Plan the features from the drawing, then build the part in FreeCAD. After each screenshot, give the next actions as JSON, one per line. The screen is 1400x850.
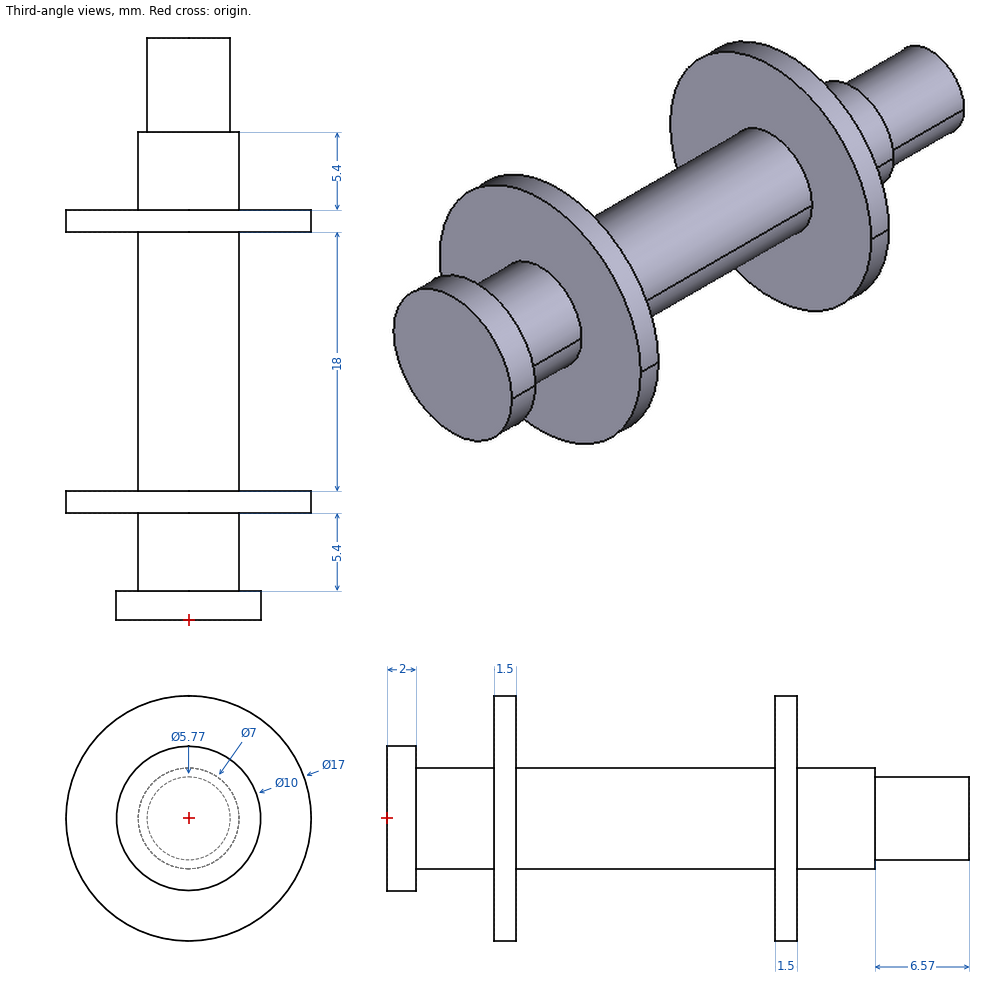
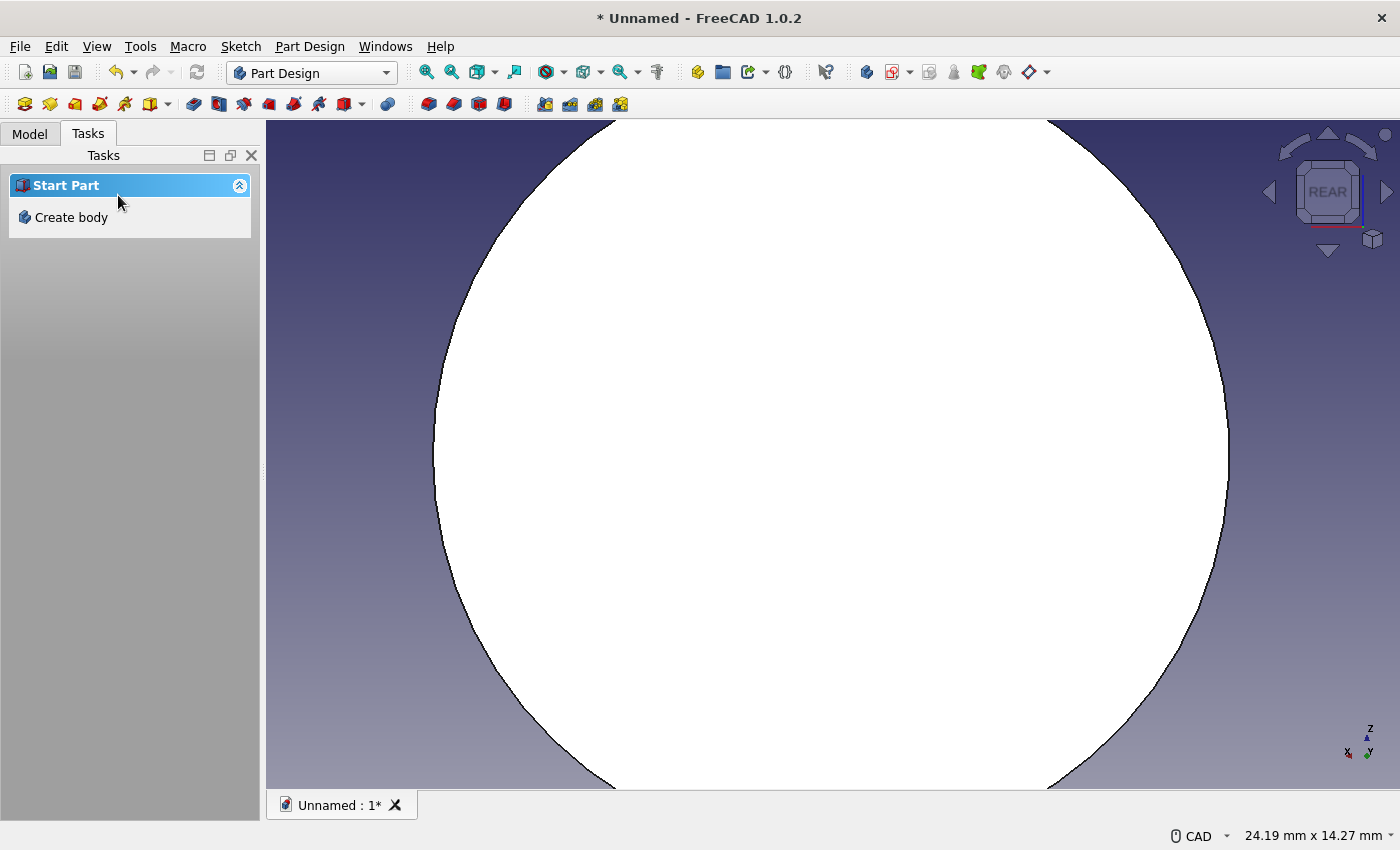
{"action": "left_click", "coordinate": [427, 72]}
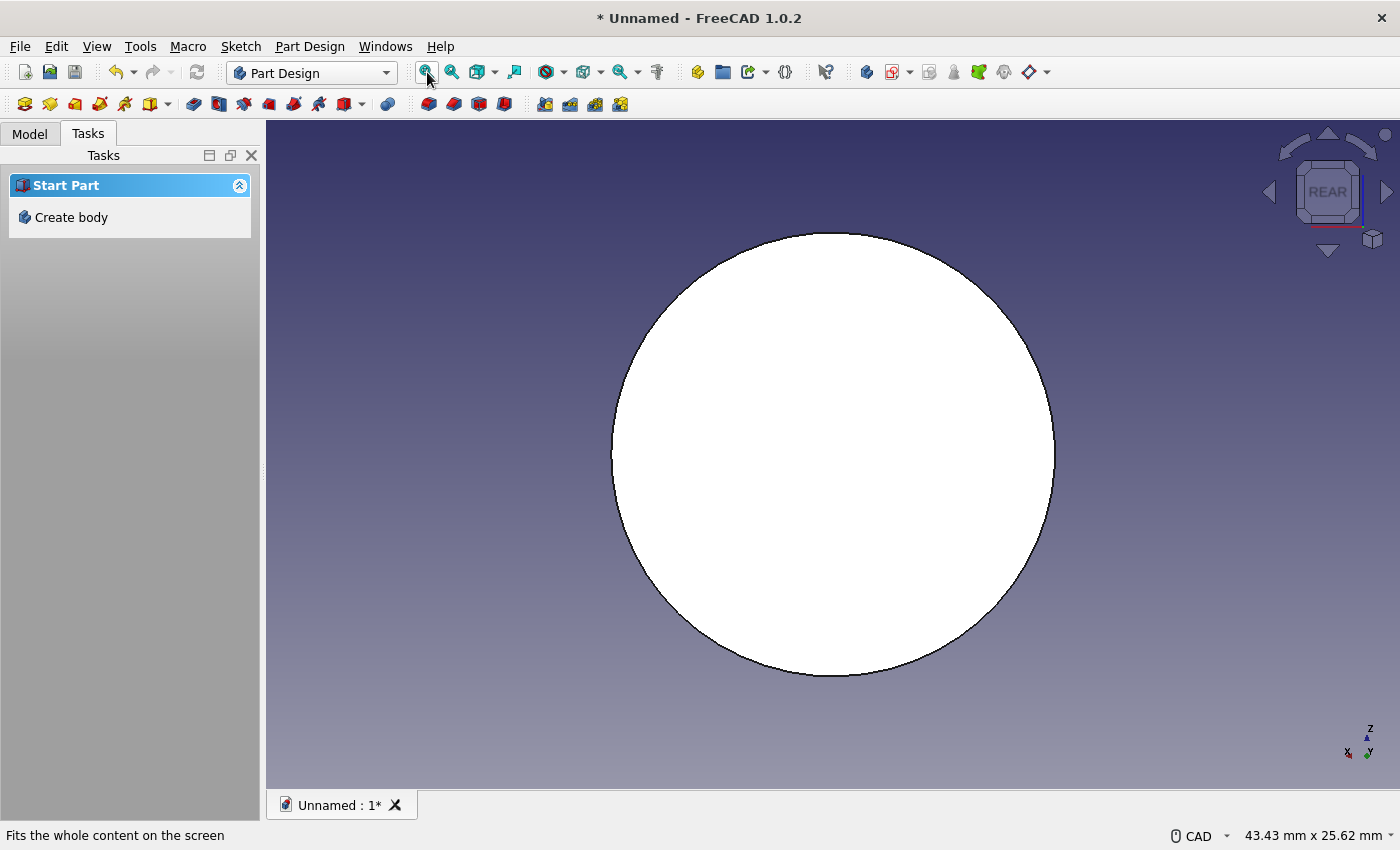
{"action": "left_click", "coordinate": [833, 453]}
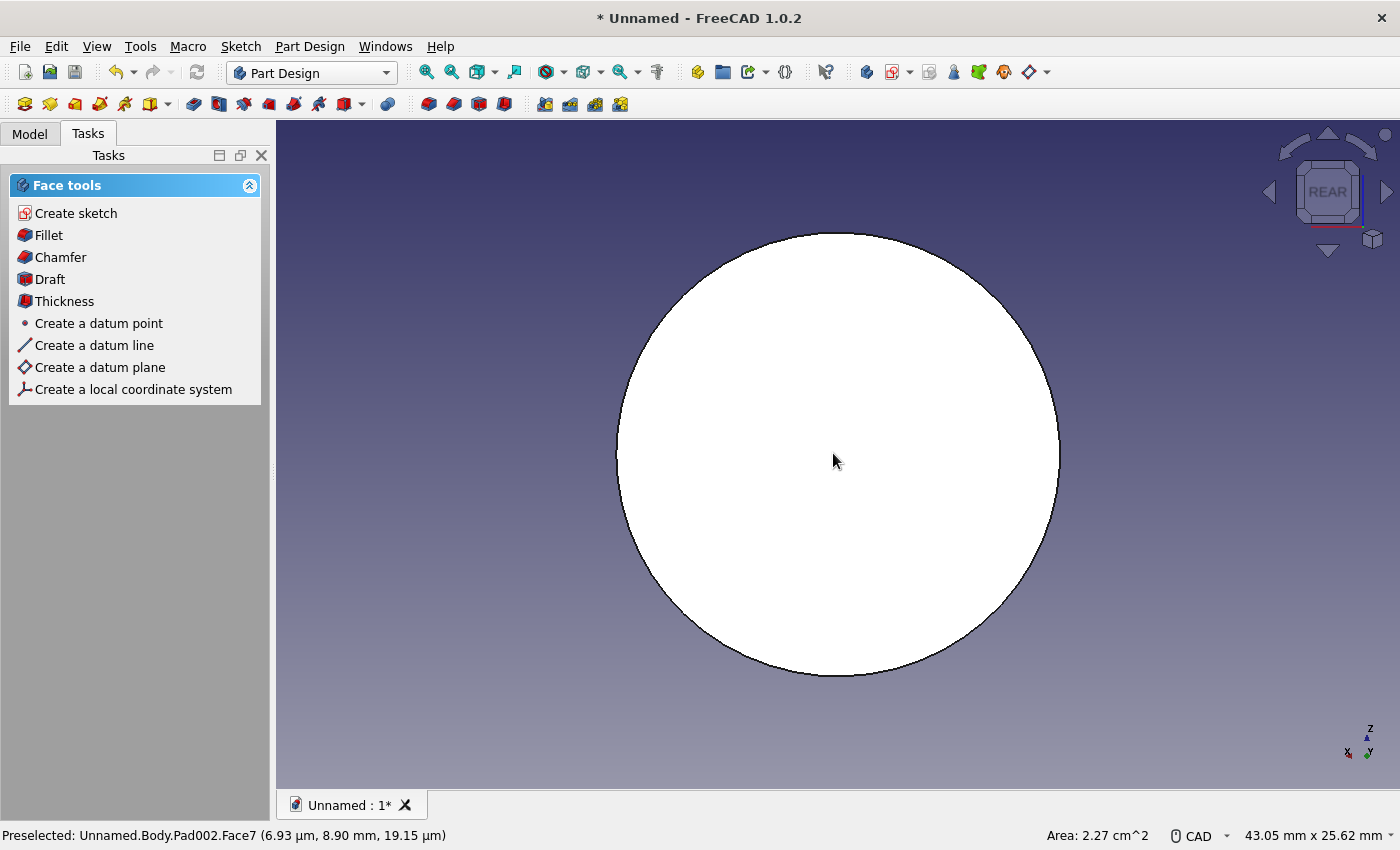
{"action": "left_click", "coordinate": [892, 72]}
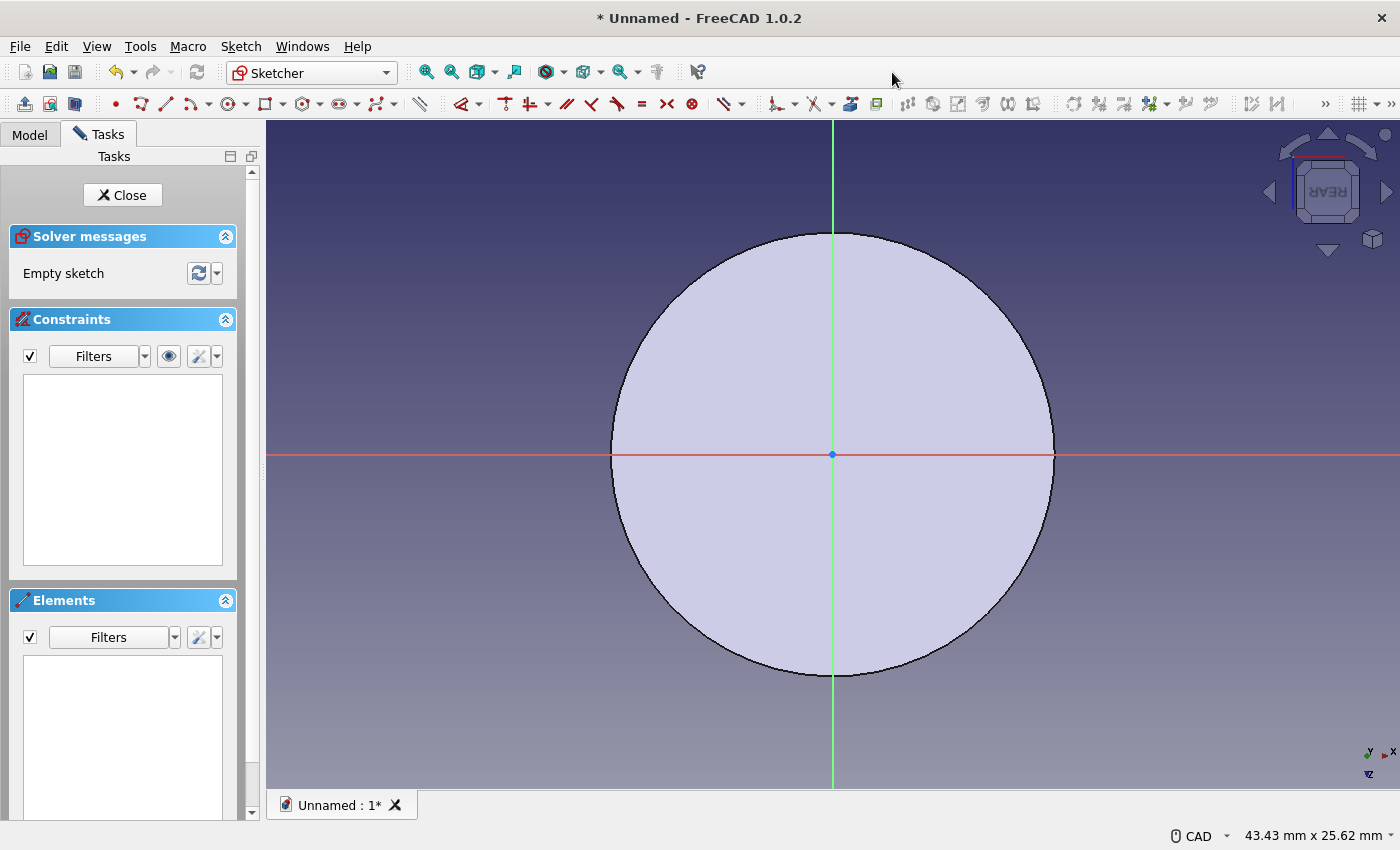
{"action": "scroll", "coordinate": [889, 454], "scroll_direction": "up", "scroll_amount": 4}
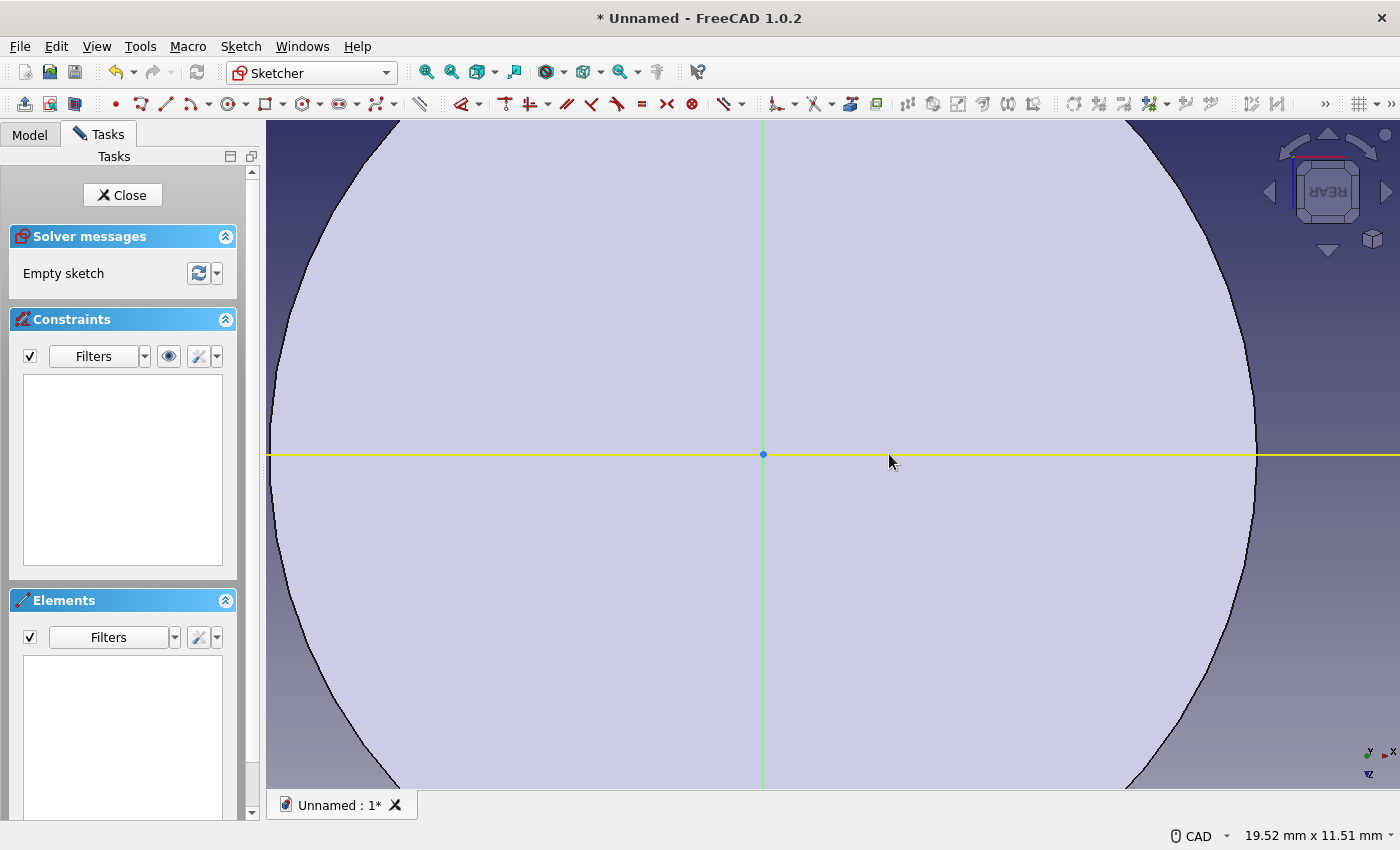
{"action": "left_click", "coordinate": [228, 104]}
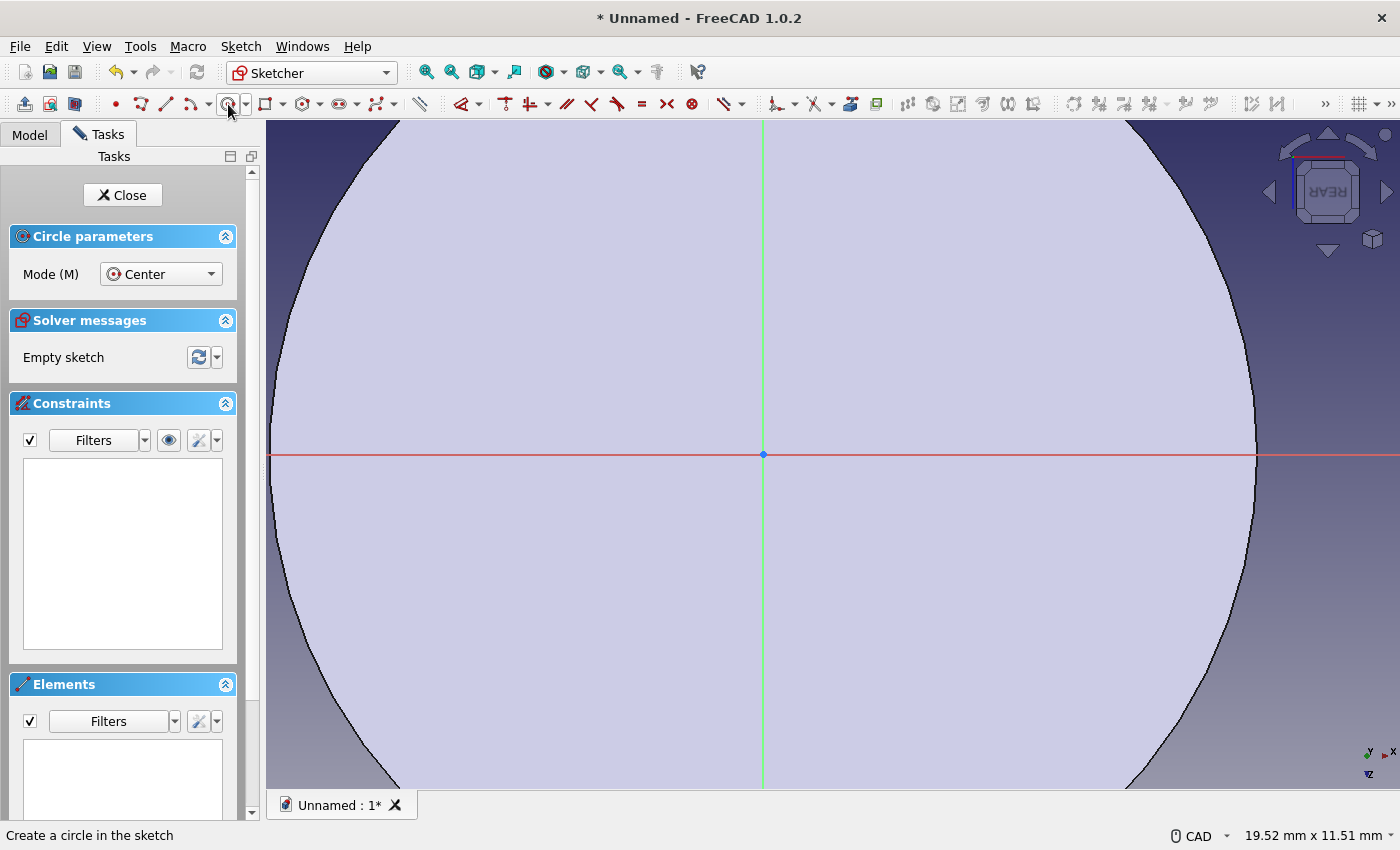
{"action": "left_click", "coordinate": [763, 454]}
{"action": "left_click", "coordinate": [907, 311]}
{"action": "key", "text": "Escape"}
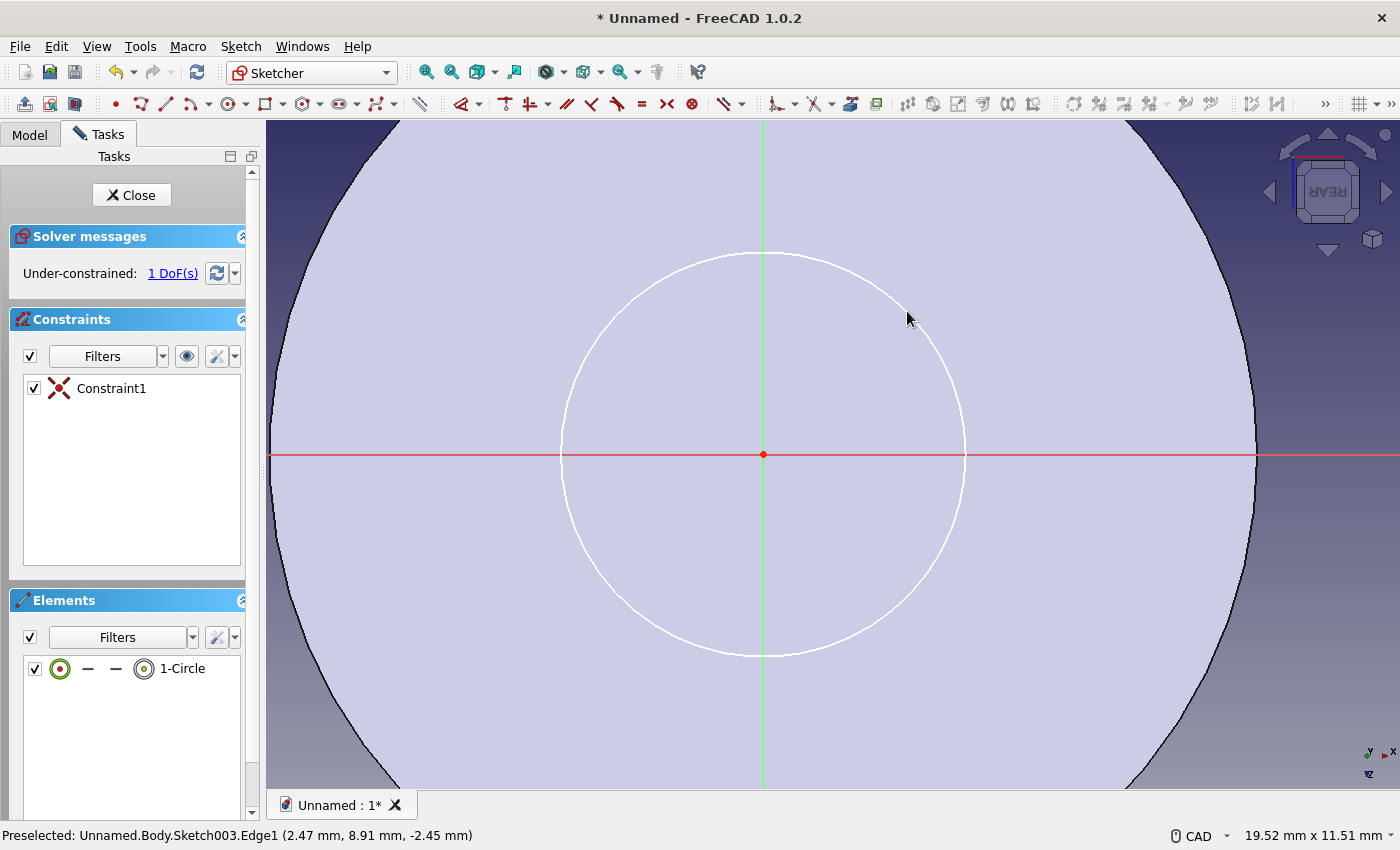
{"action": "left_click", "coordinate": [460, 104]}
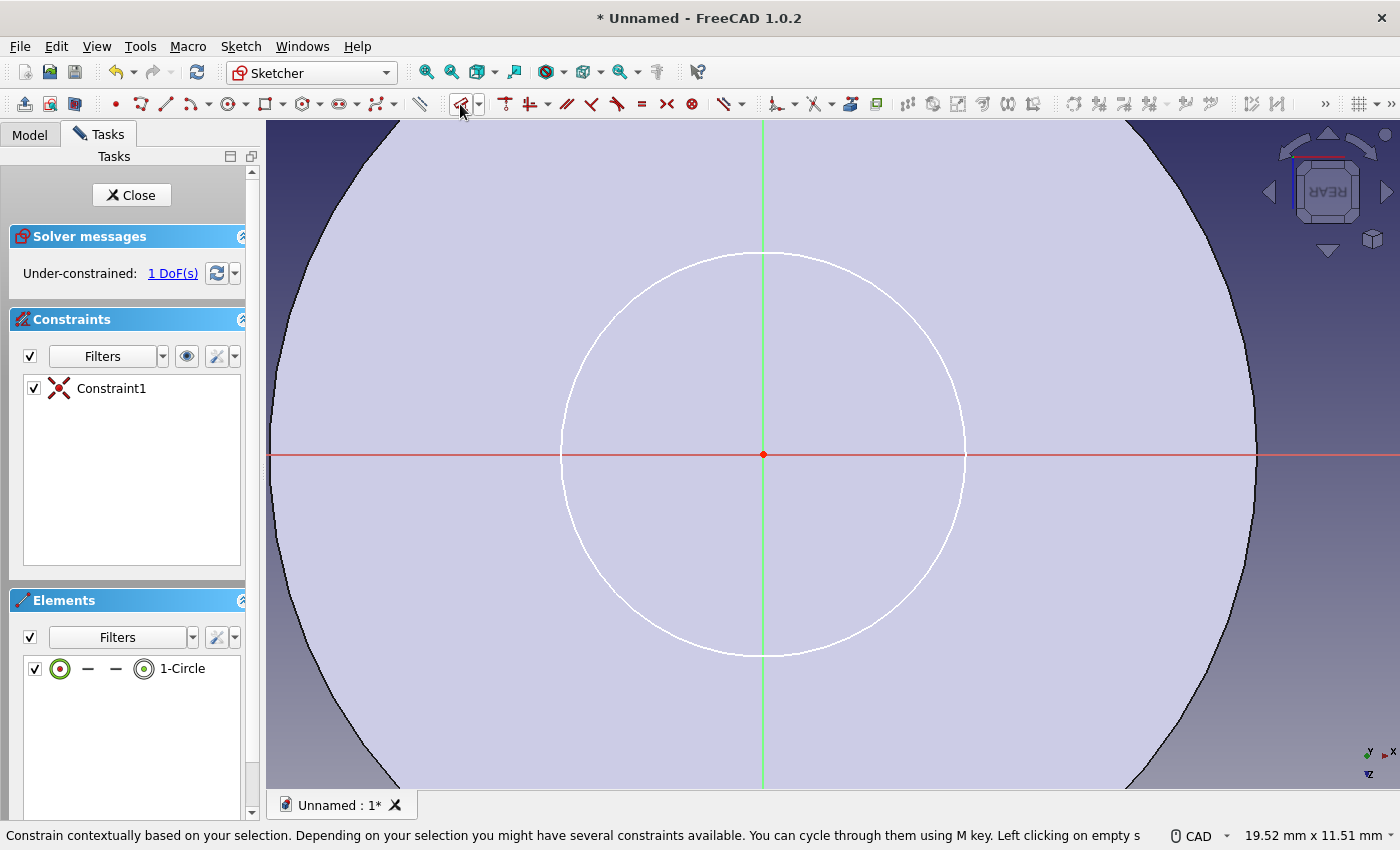
{"action": "left_click", "coordinate": [906, 311]}
{"action": "left_click", "coordinate": [929, 288]}